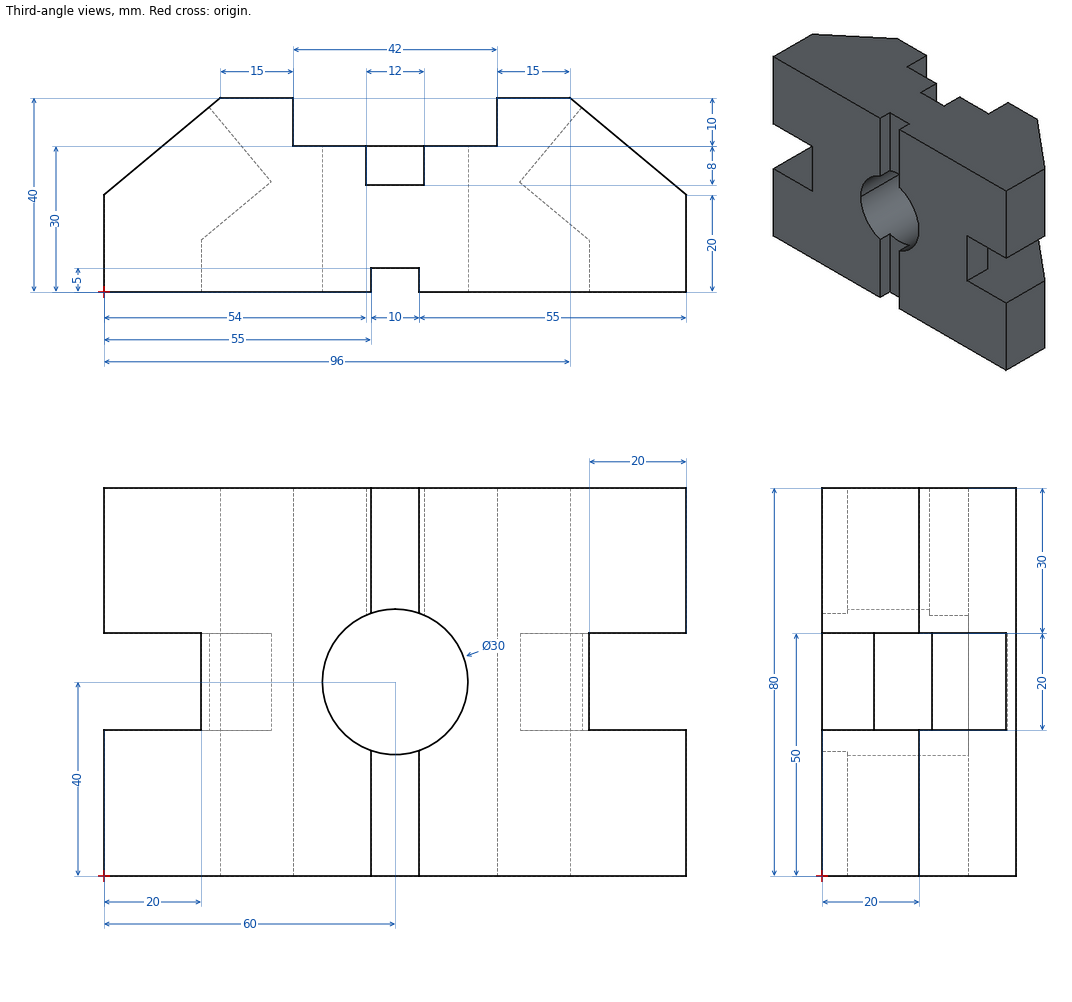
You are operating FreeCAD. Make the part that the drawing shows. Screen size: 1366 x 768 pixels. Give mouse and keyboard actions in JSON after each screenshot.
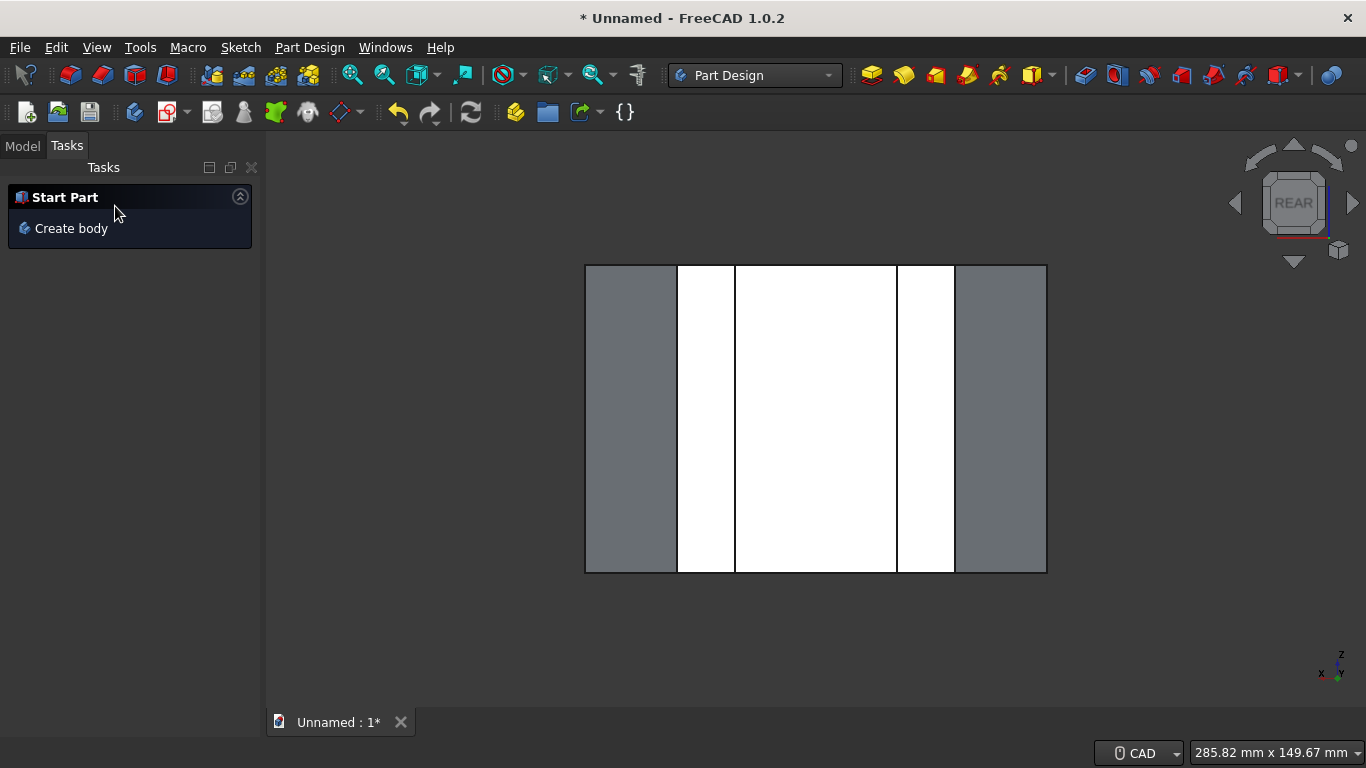
{"action": "left_click", "coordinate": [816, 374]}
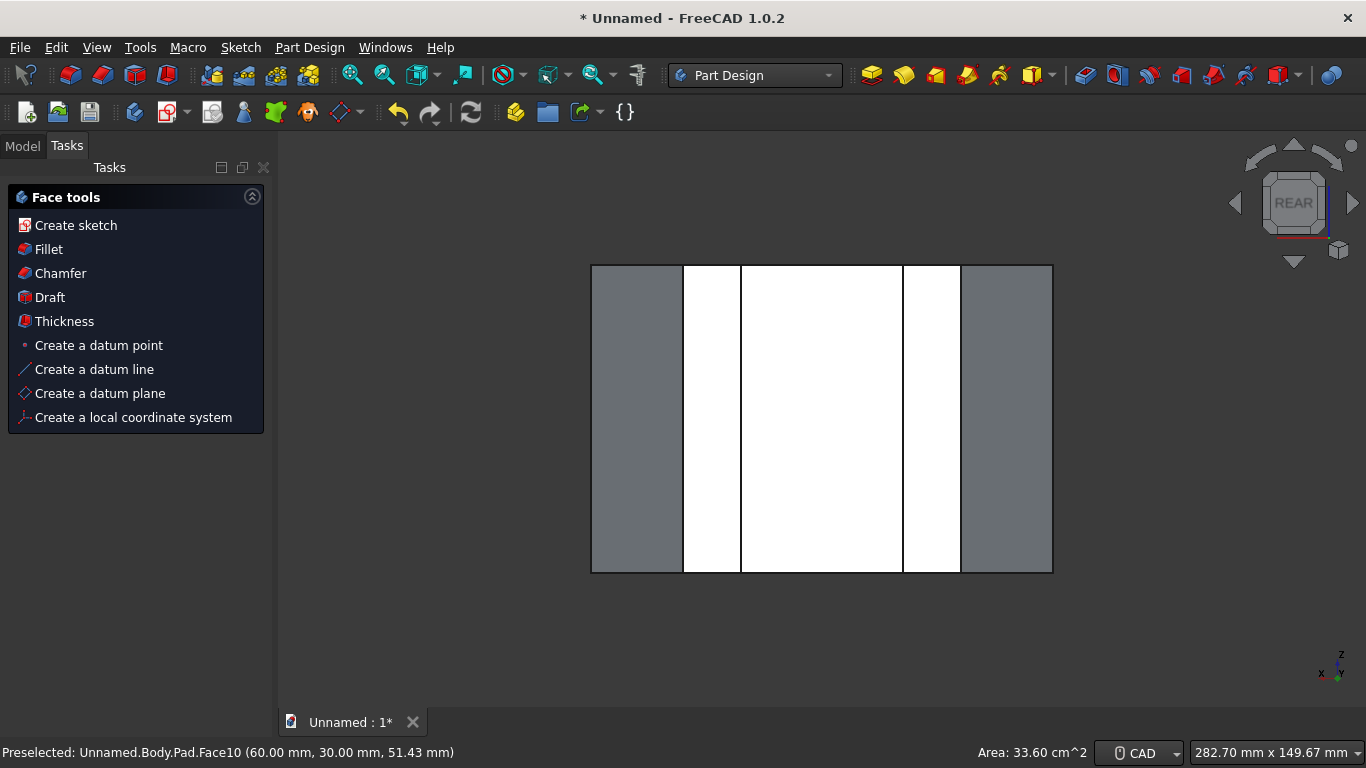
{"action": "left_click", "coordinate": [168, 112]}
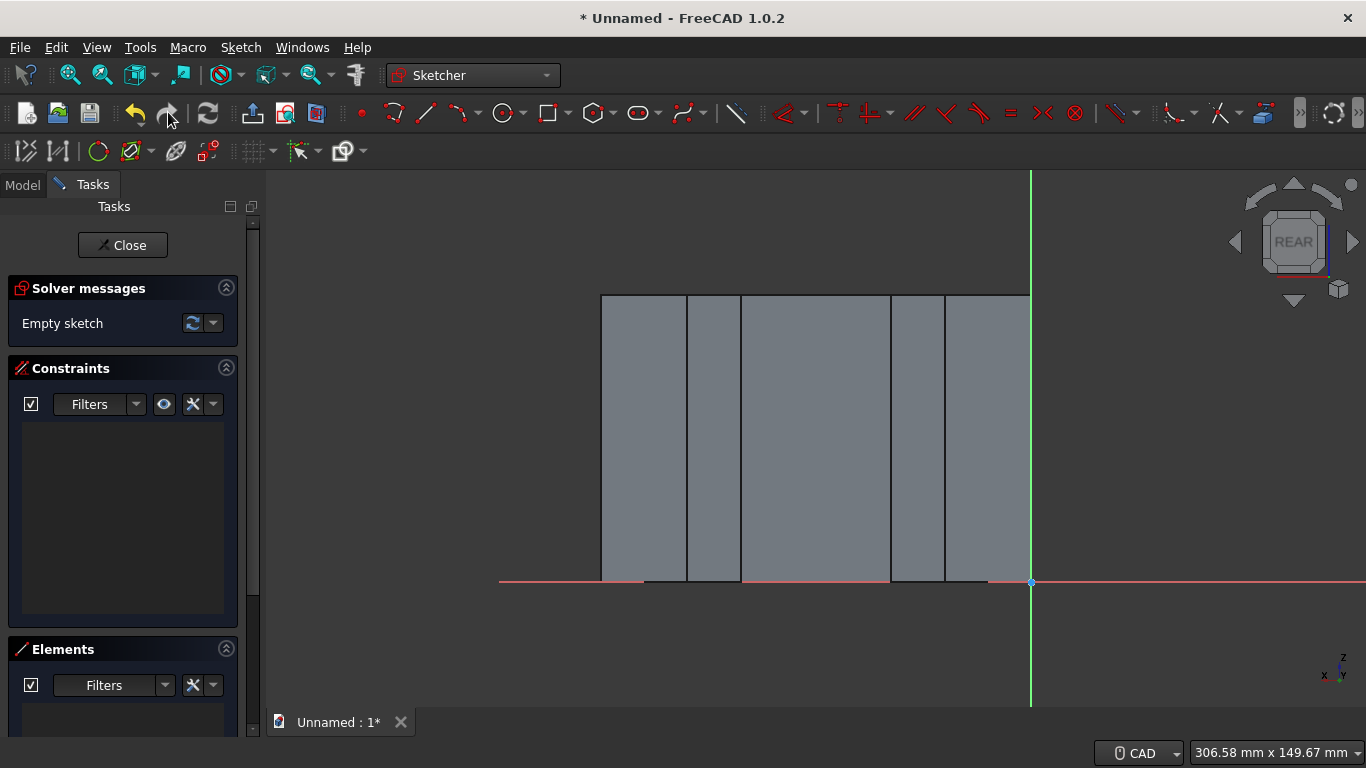
{"action": "scroll", "coordinate": [846, 438], "scroll_direction": "up", "scroll_amount": 6}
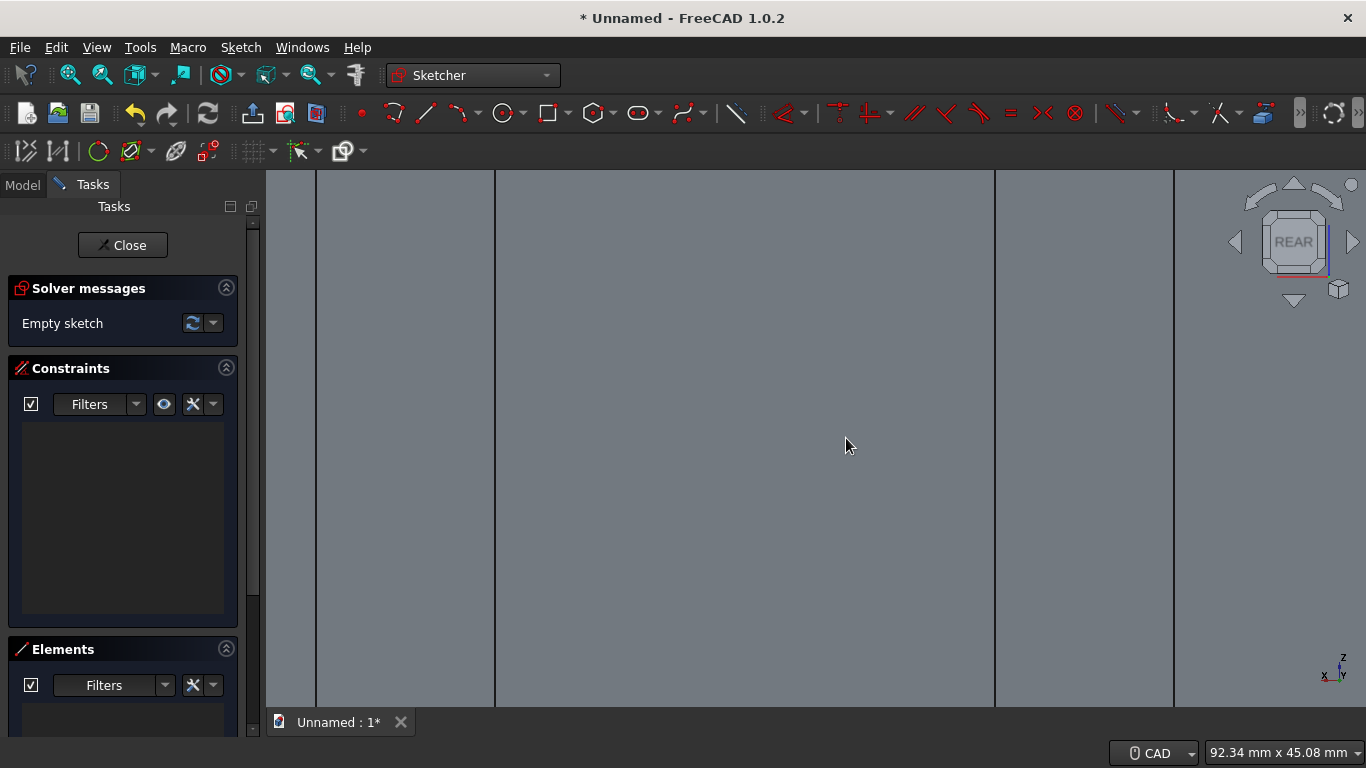
{"action": "key", "text": "g c"}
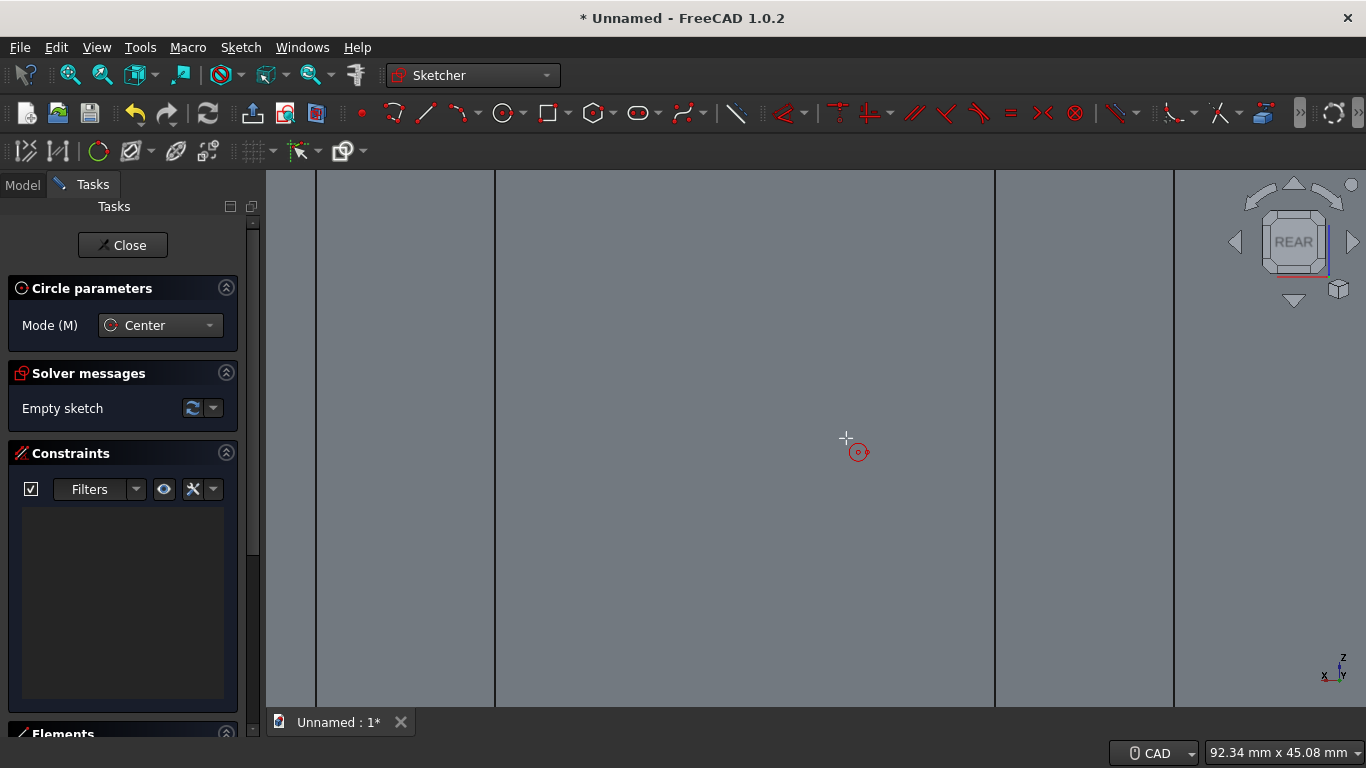
{"action": "left_click", "coordinate": [745, 438]}
{"action": "mouse_move", "coordinate": [872, 312]}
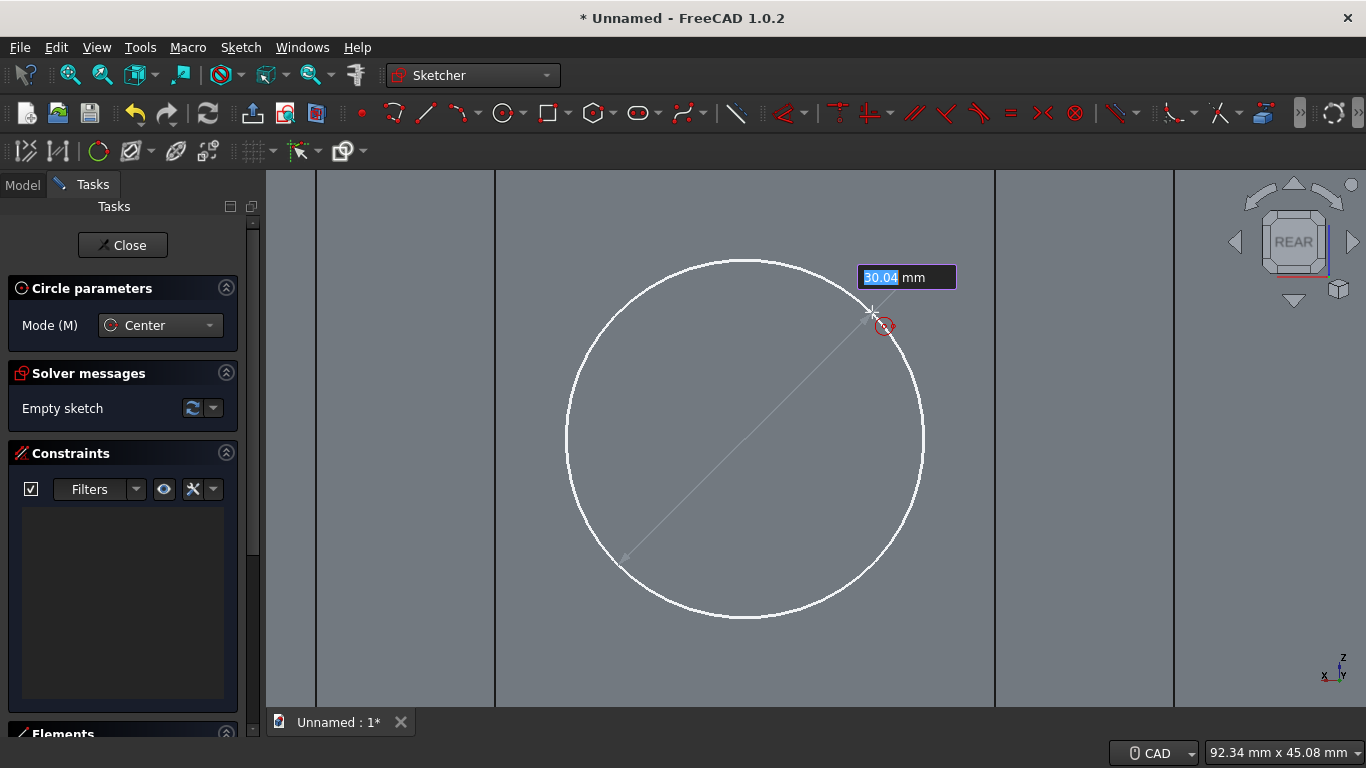
{"action": "type", "text": "30"}
{"action": "key", "text": "Return"}
{"action": "key", "text": "Escape"}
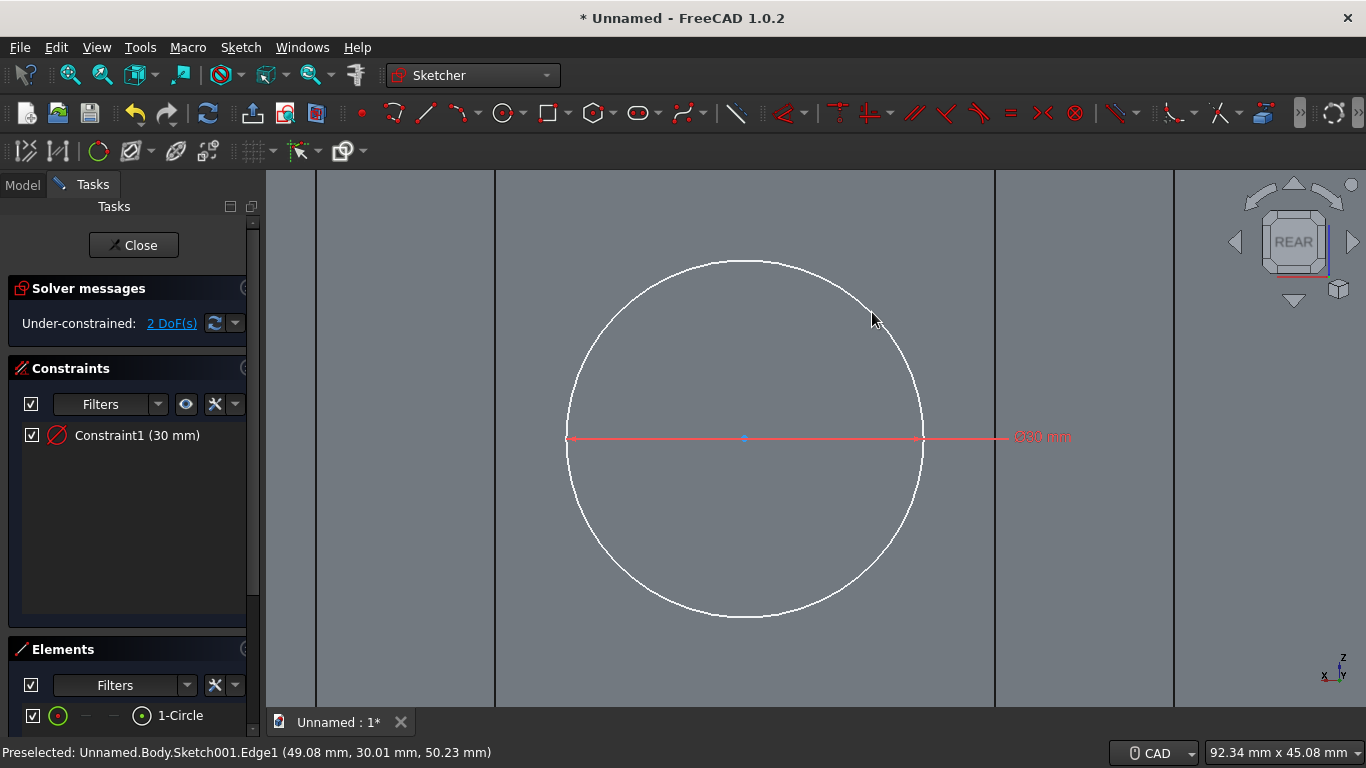
{"action": "key", "text": "d"}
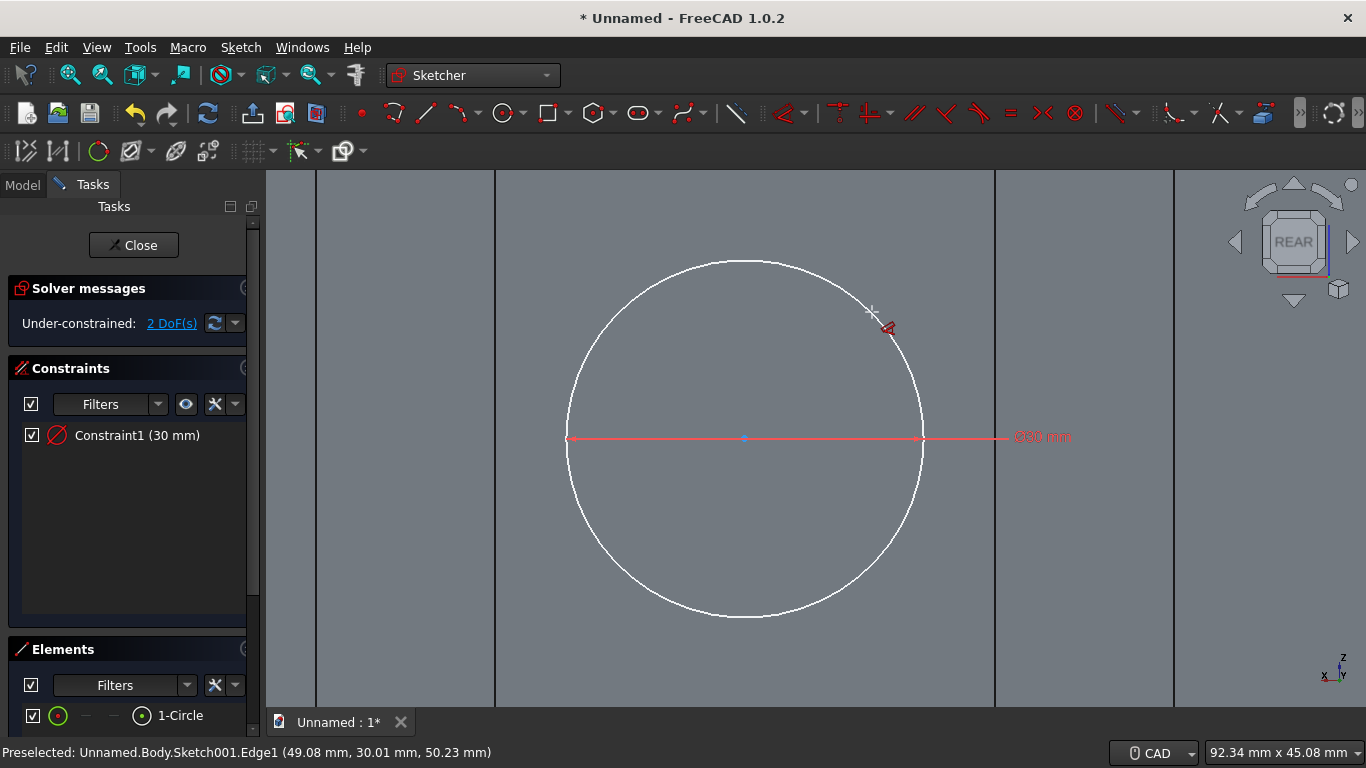
{"action": "left_click", "coordinate": [745, 439]}
{"action": "left_click", "coordinate": [973, 405]}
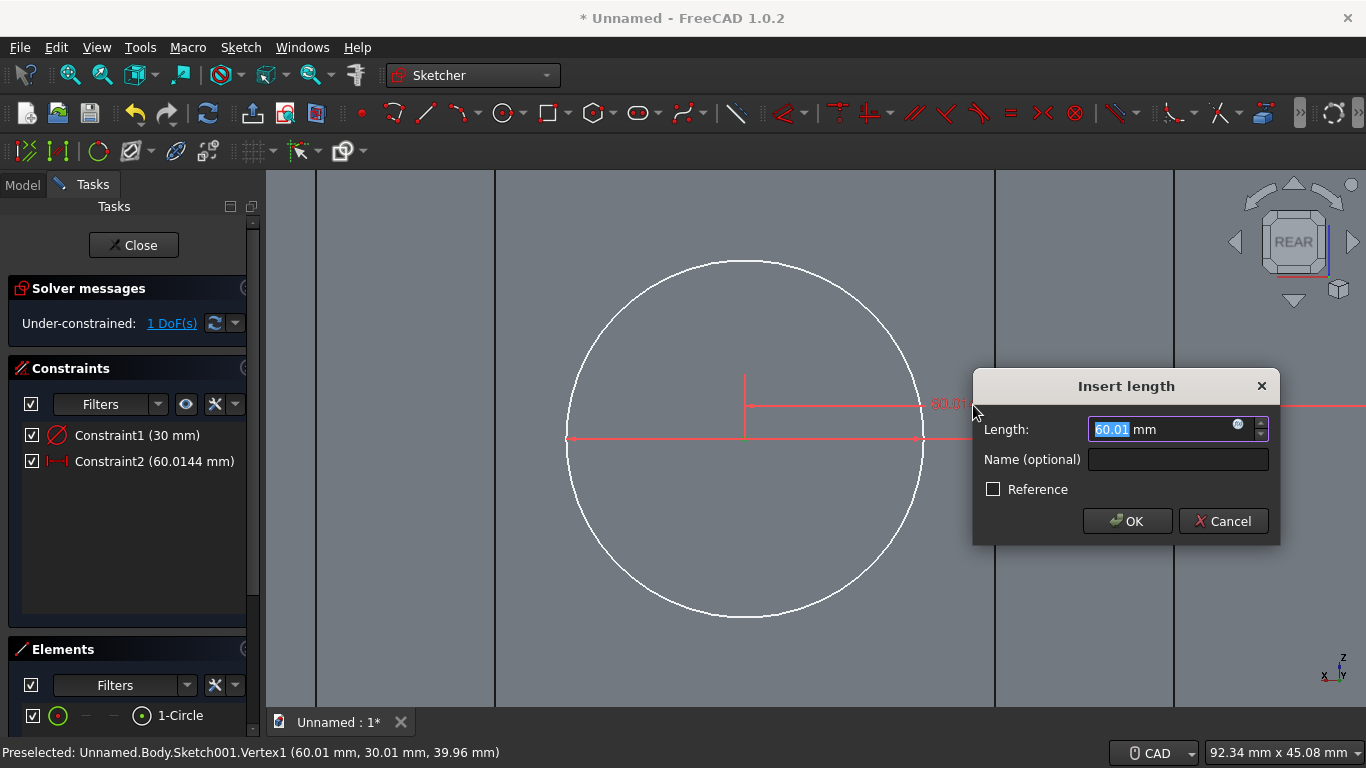
{"action": "type", "text": "60"}
{"action": "key", "text": "Return"}